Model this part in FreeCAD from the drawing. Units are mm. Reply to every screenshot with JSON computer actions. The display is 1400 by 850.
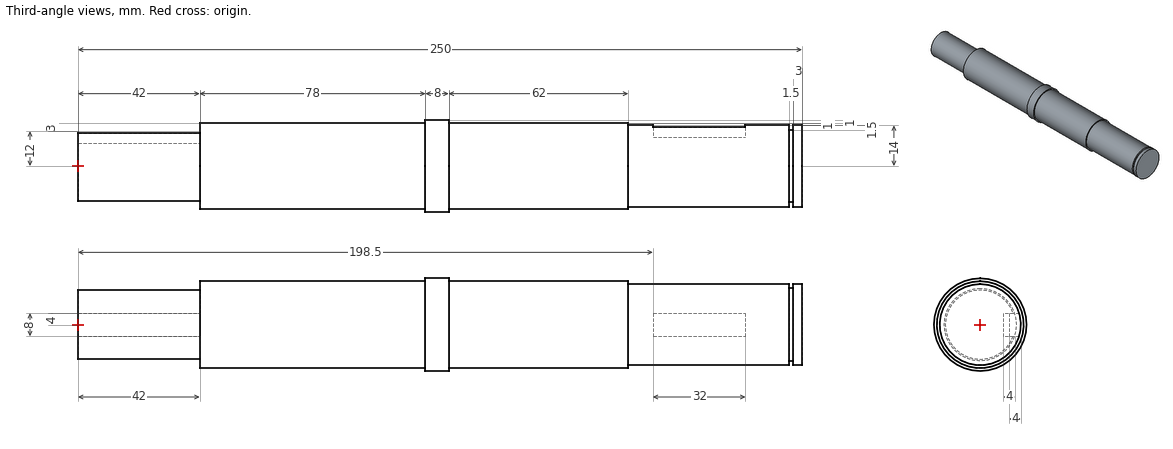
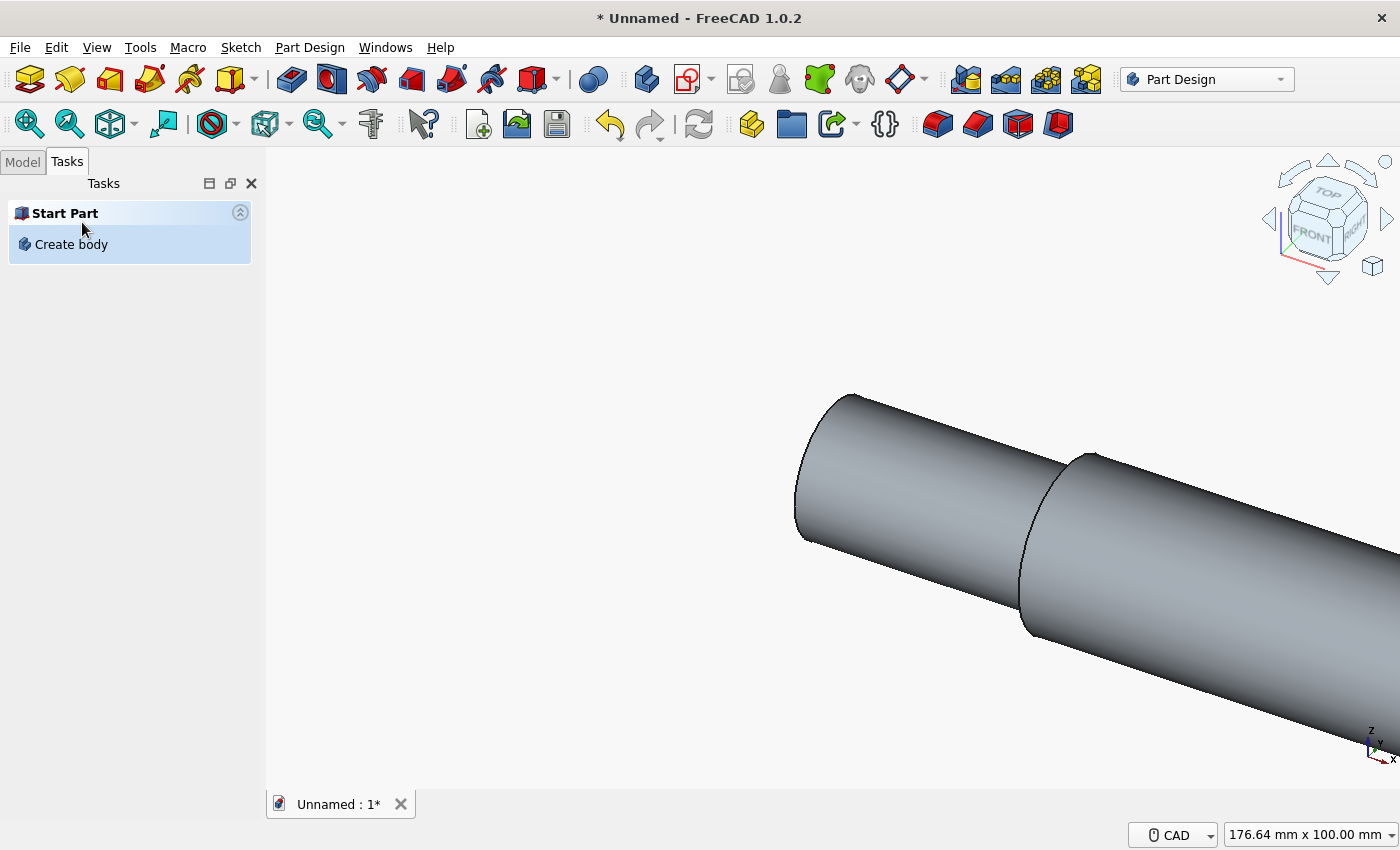
{"action": "left_click", "coordinate": [30, 124]}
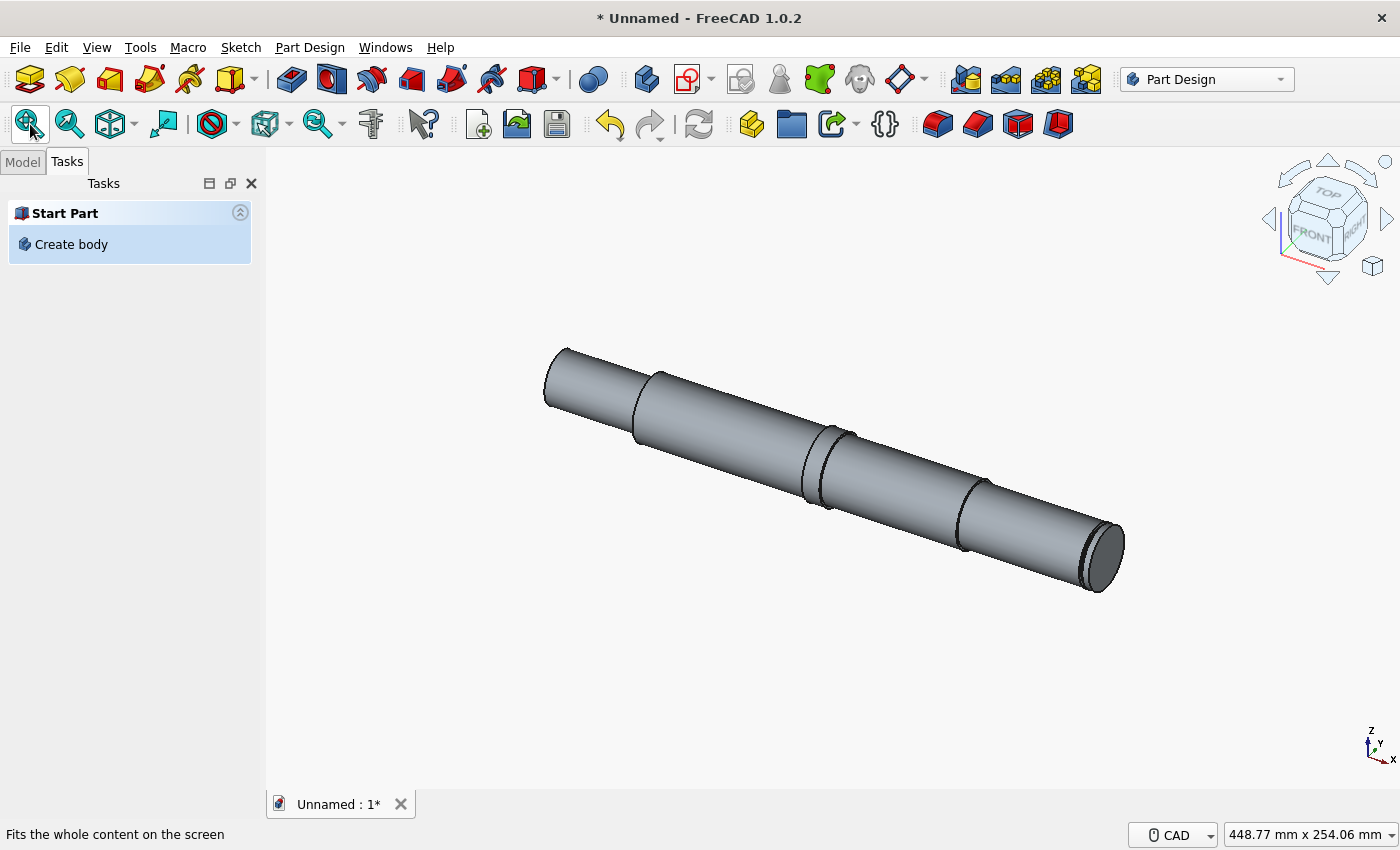
{"action": "left_click", "coordinate": [23, 161]}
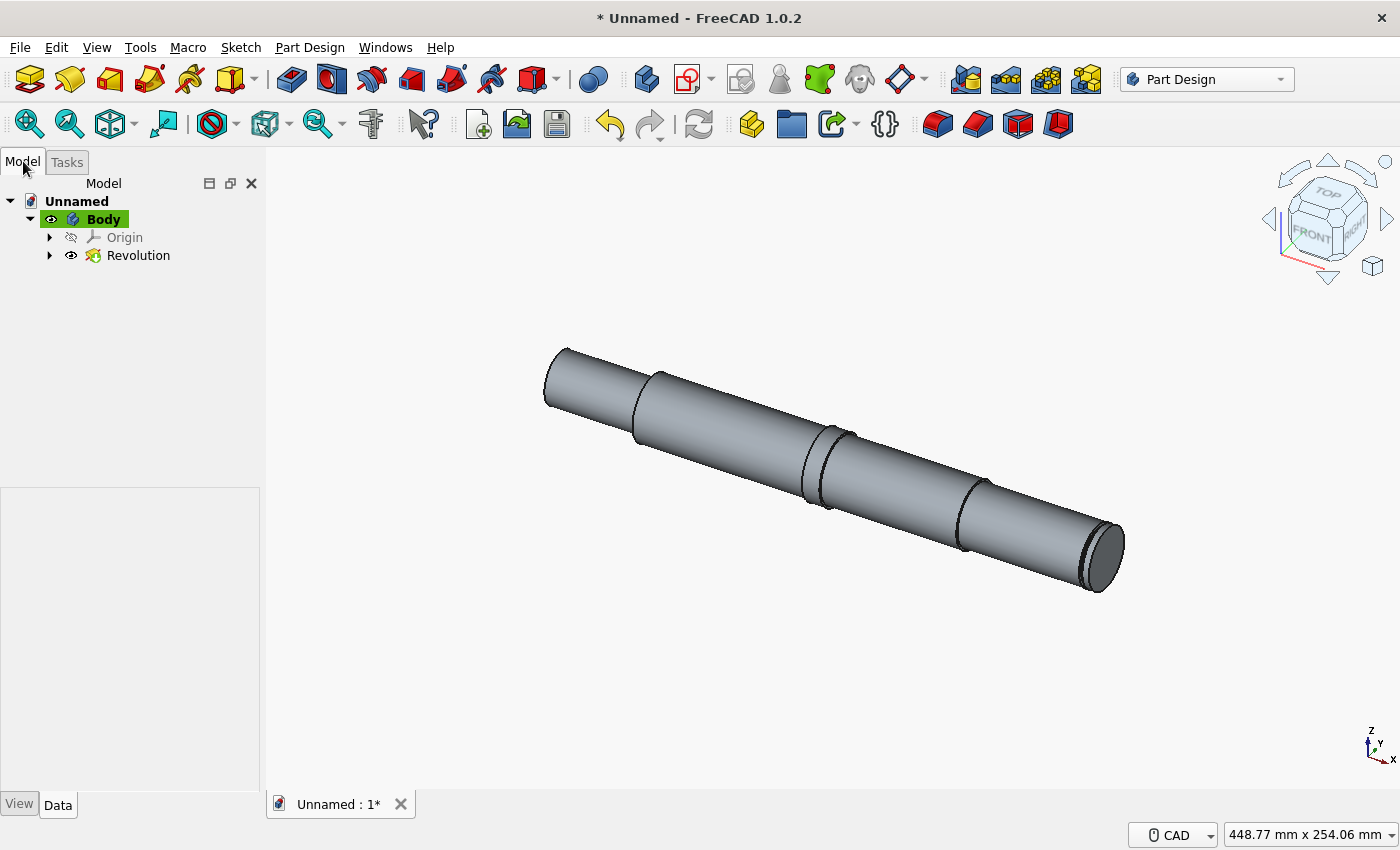
{"action": "left_click", "coordinate": [50, 237]}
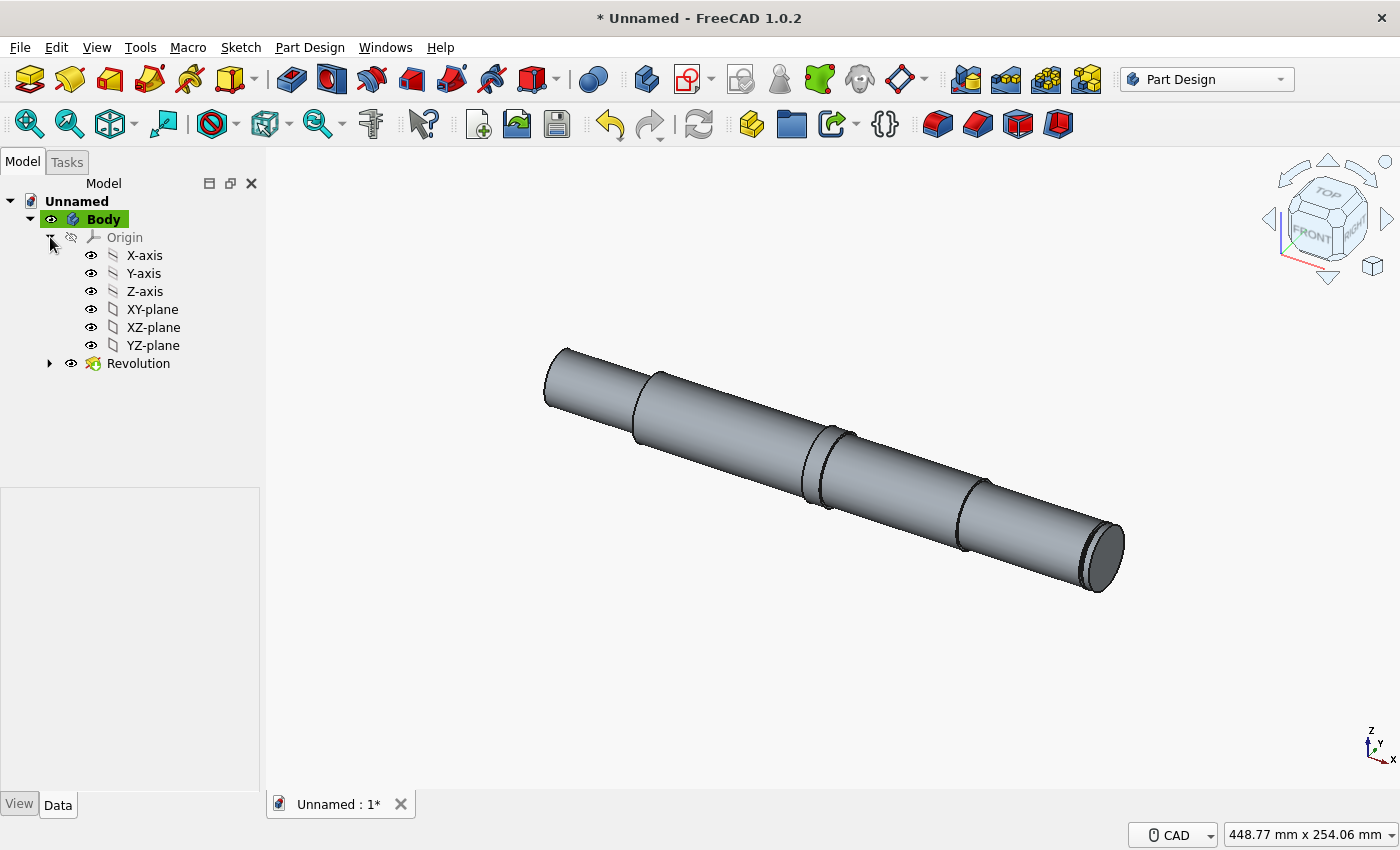
{"action": "left_click", "coordinate": [136, 327]}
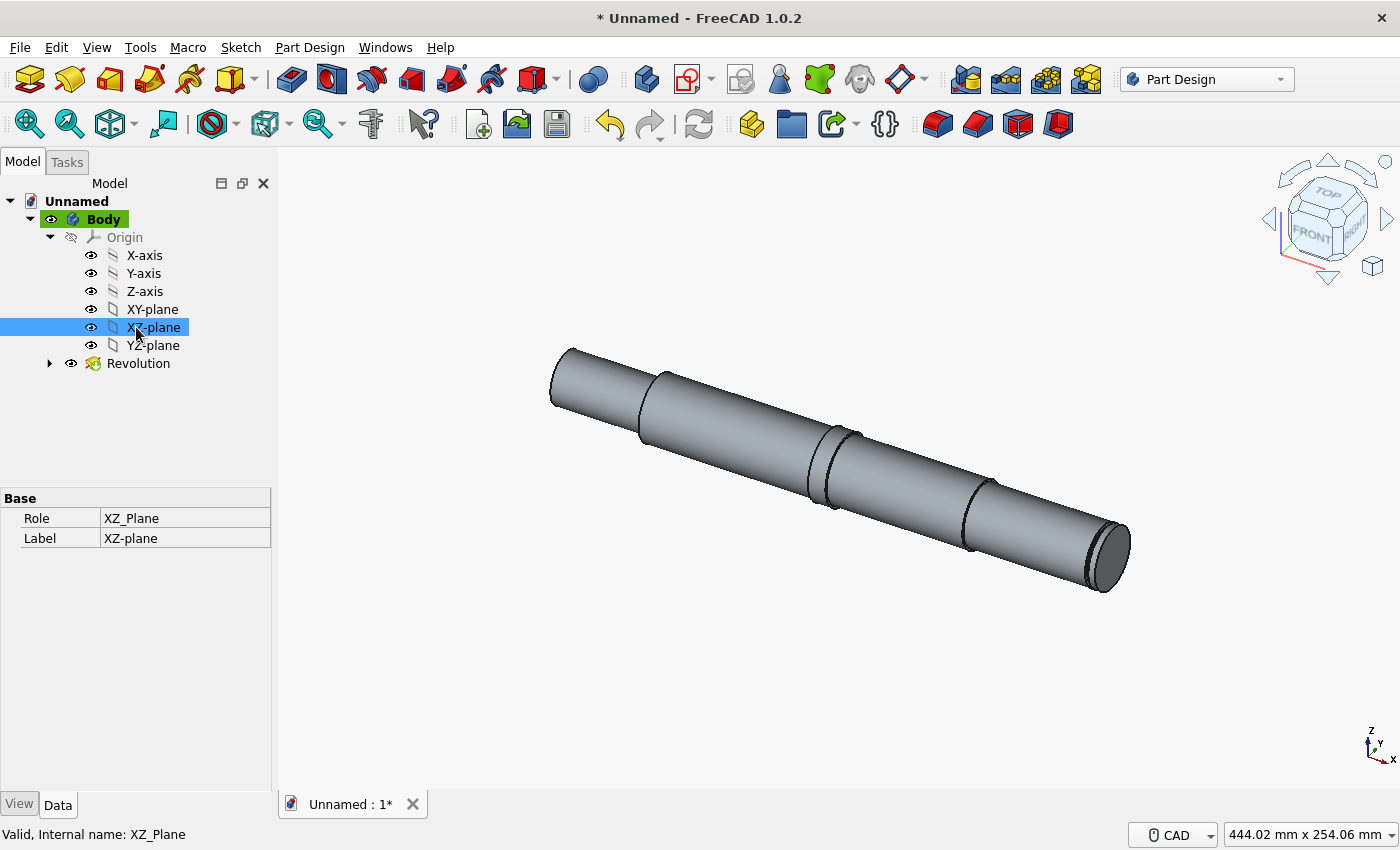
{"action": "left_click", "coordinate": [900, 80]}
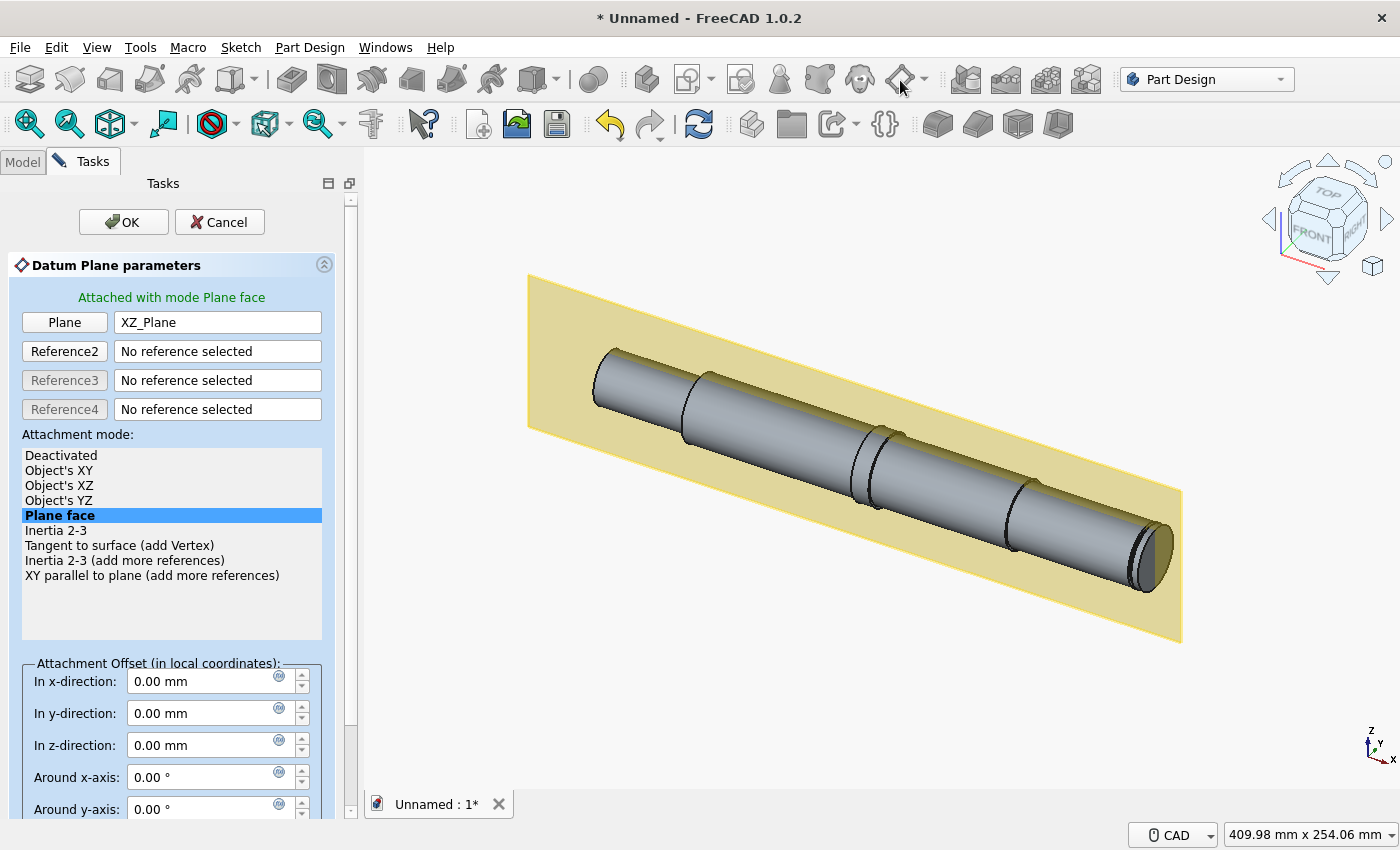
{"action": "triple_click", "coordinate": [210, 745]}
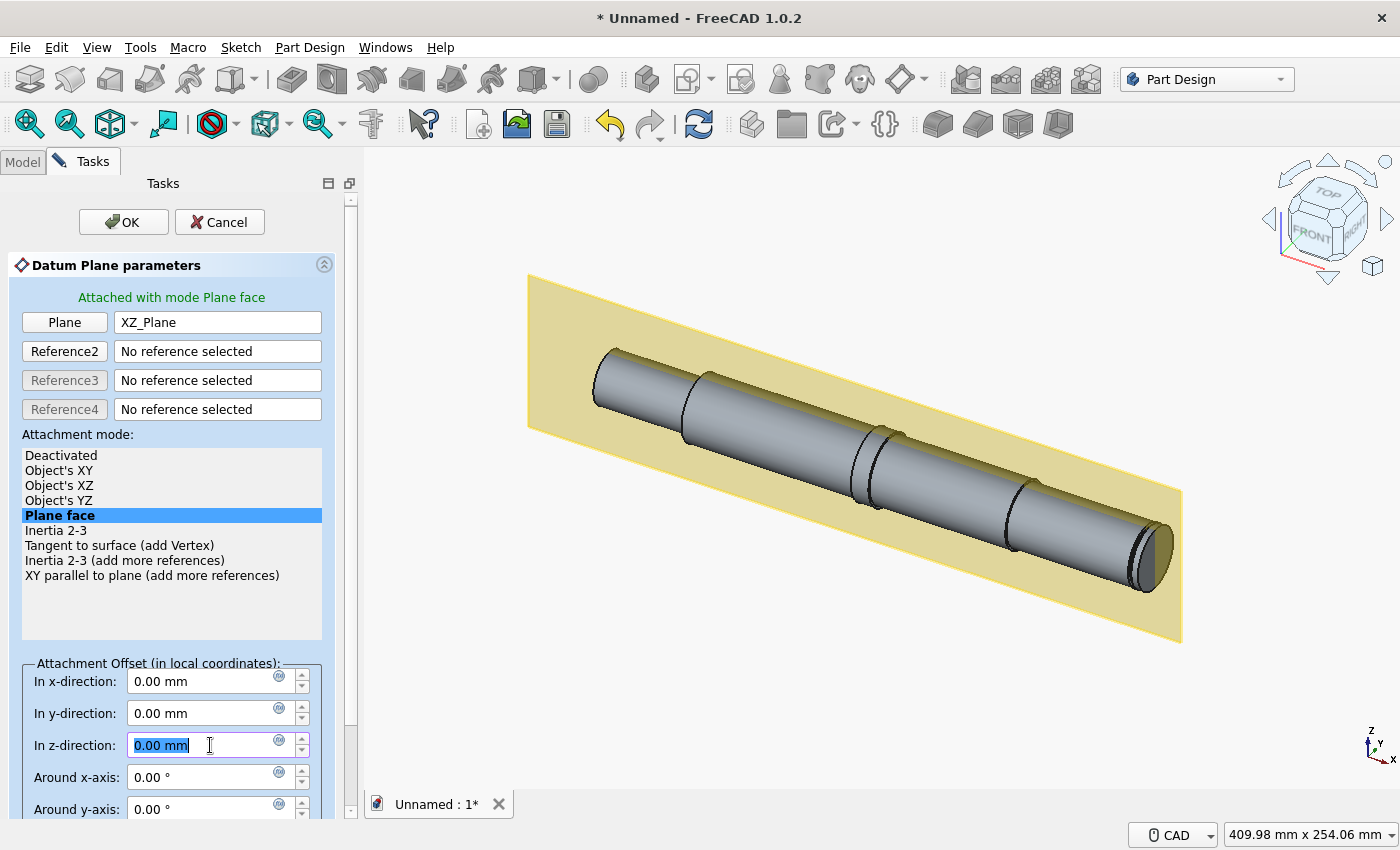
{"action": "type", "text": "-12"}
{"action": "key", "text": "Tab"}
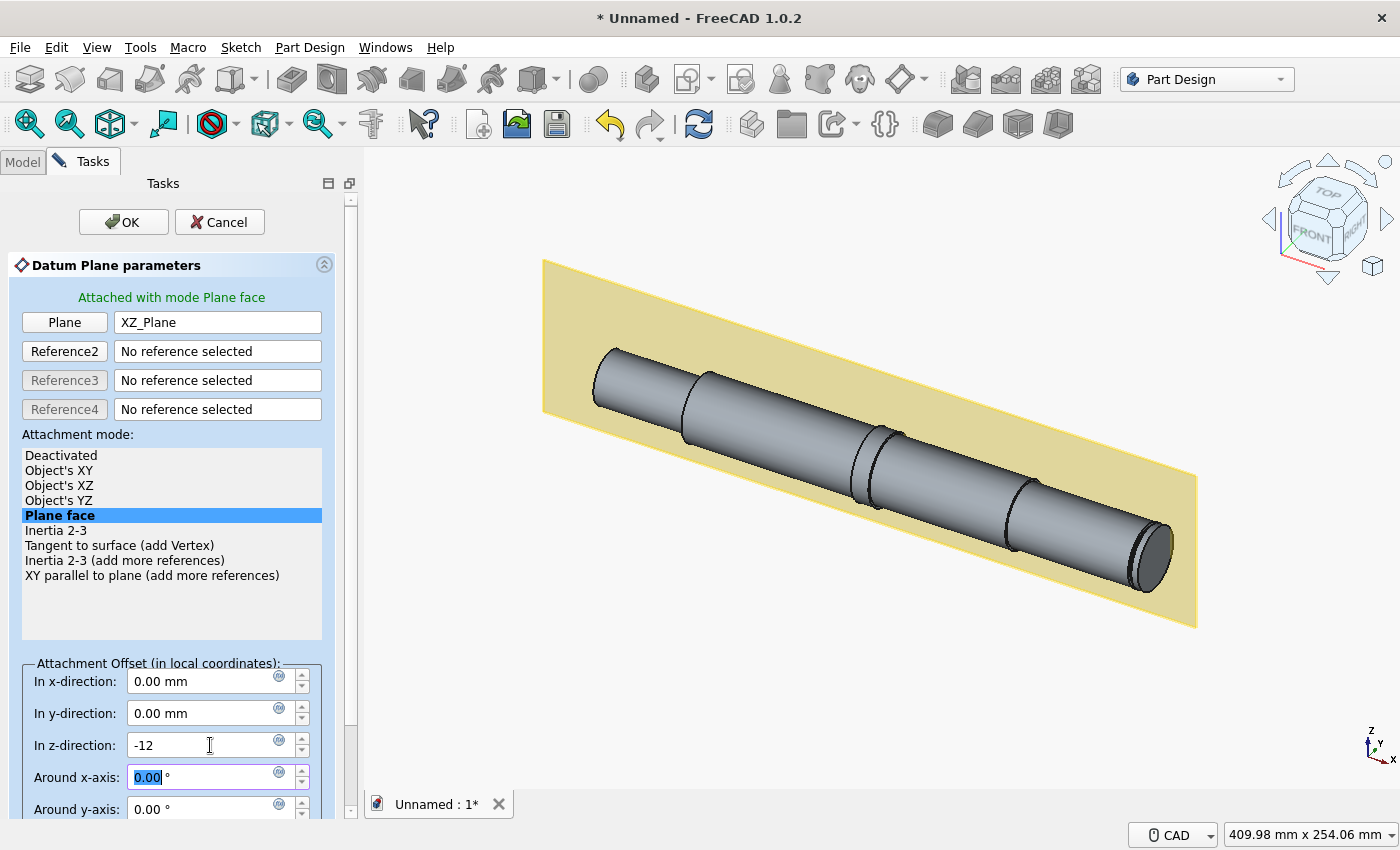
{"action": "left_click", "coordinate": [124, 222]}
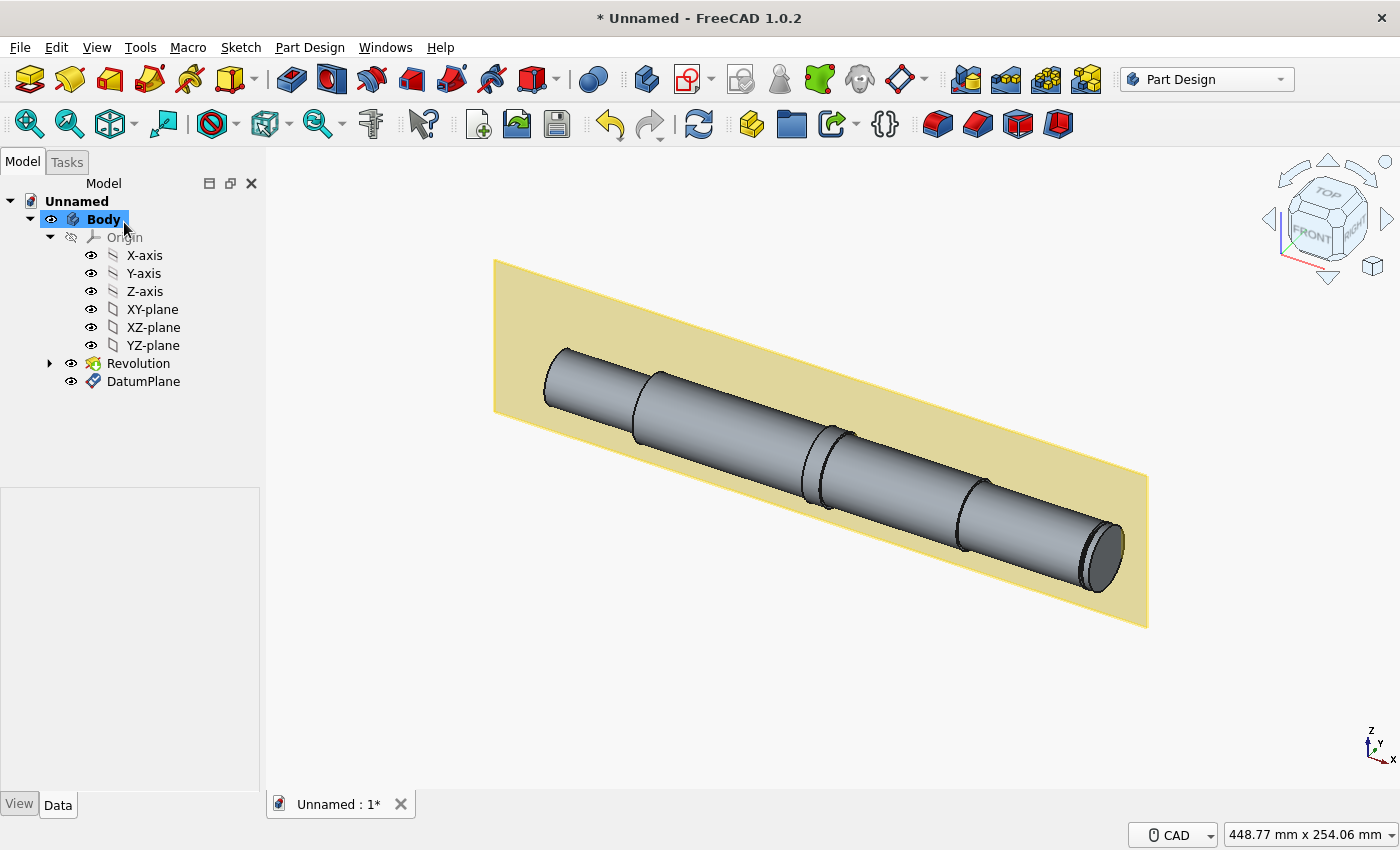
{"action": "left_click", "coordinate": [116, 381]}